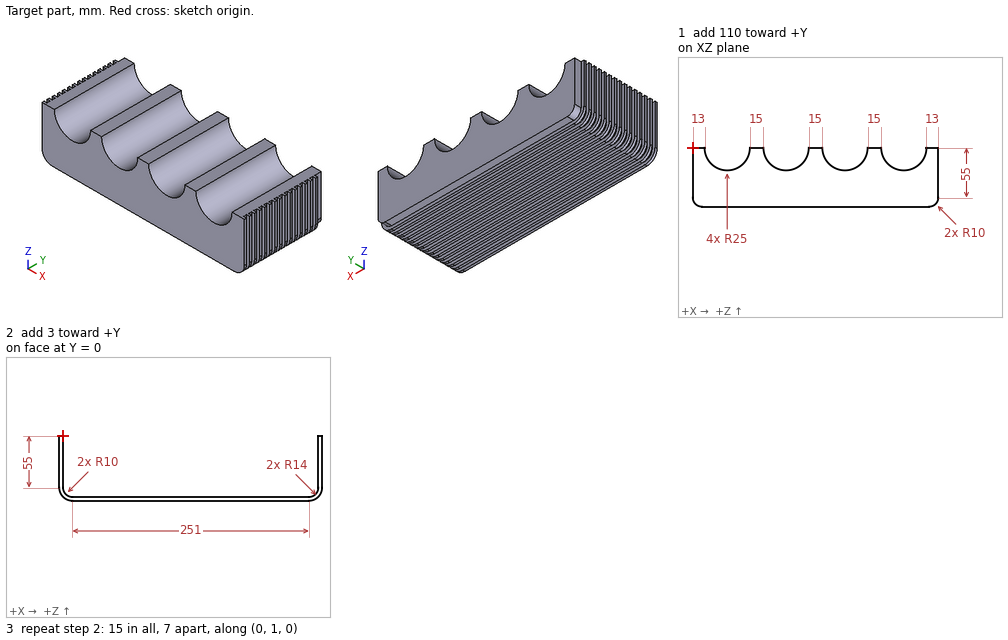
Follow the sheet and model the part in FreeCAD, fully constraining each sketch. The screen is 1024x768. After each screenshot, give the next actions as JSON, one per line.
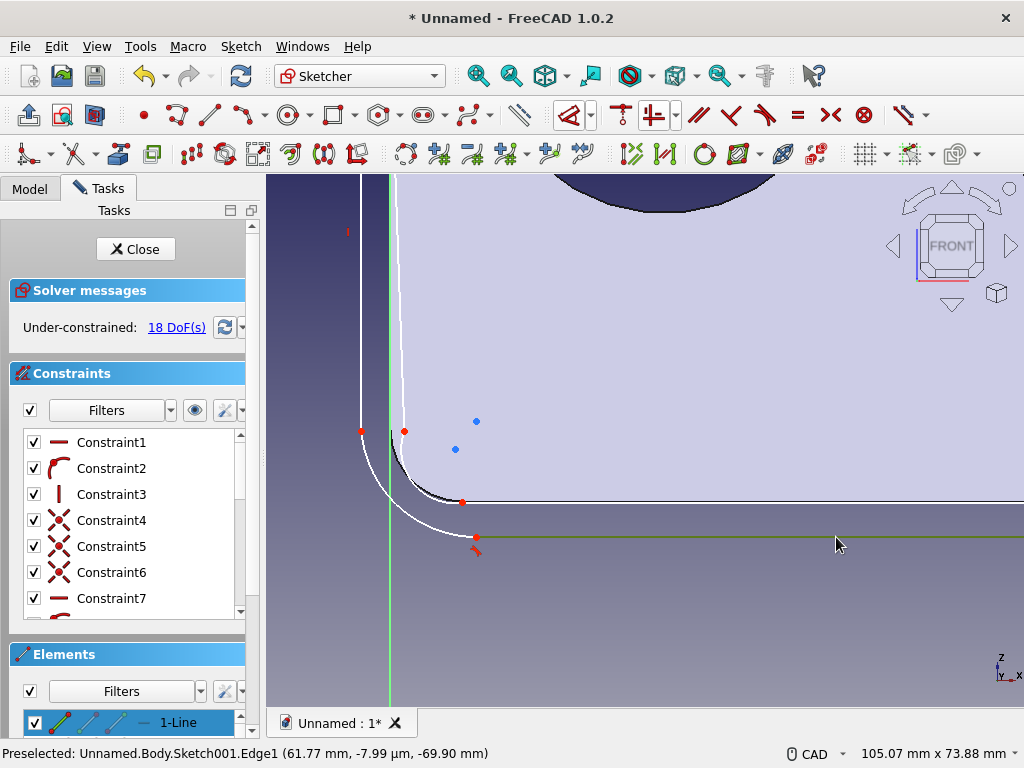
{"action": "scroll", "coordinate": [376, 481], "scroll_direction": "down", "scroll_amount": 8}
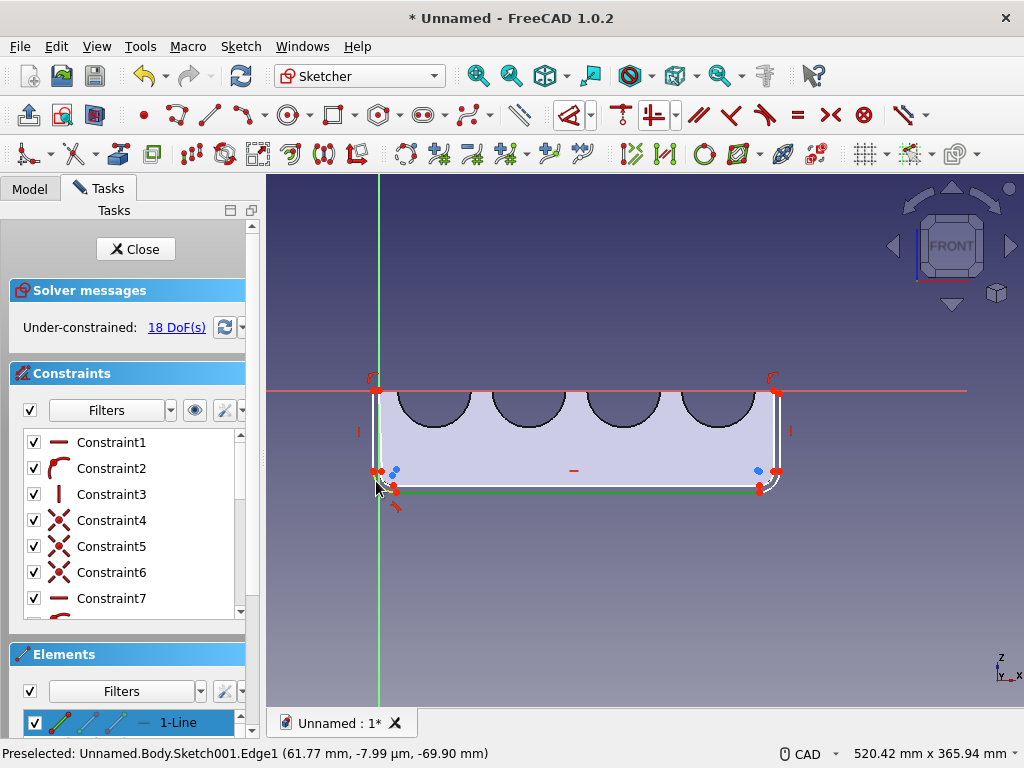
{"action": "scroll", "coordinate": [768, 490], "scroll_direction": "up", "scroll_amount": 5}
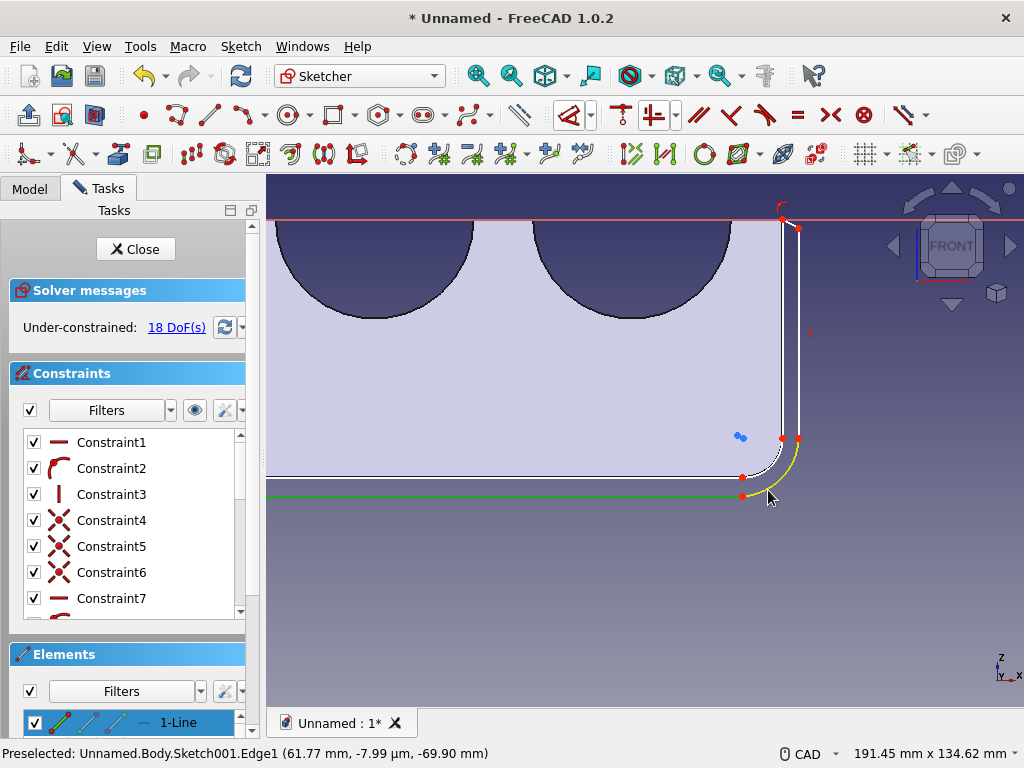
{"action": "left_click", "coordinate": [768, 489]}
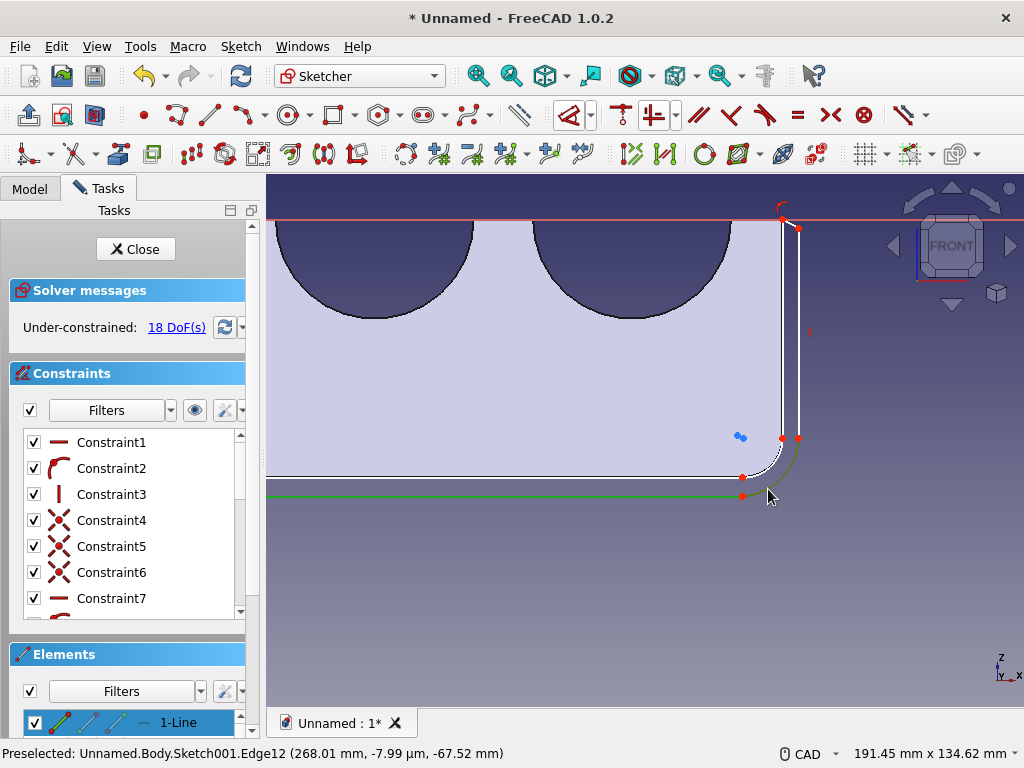
{"action": "left_click", "coordinate": [765, 116]}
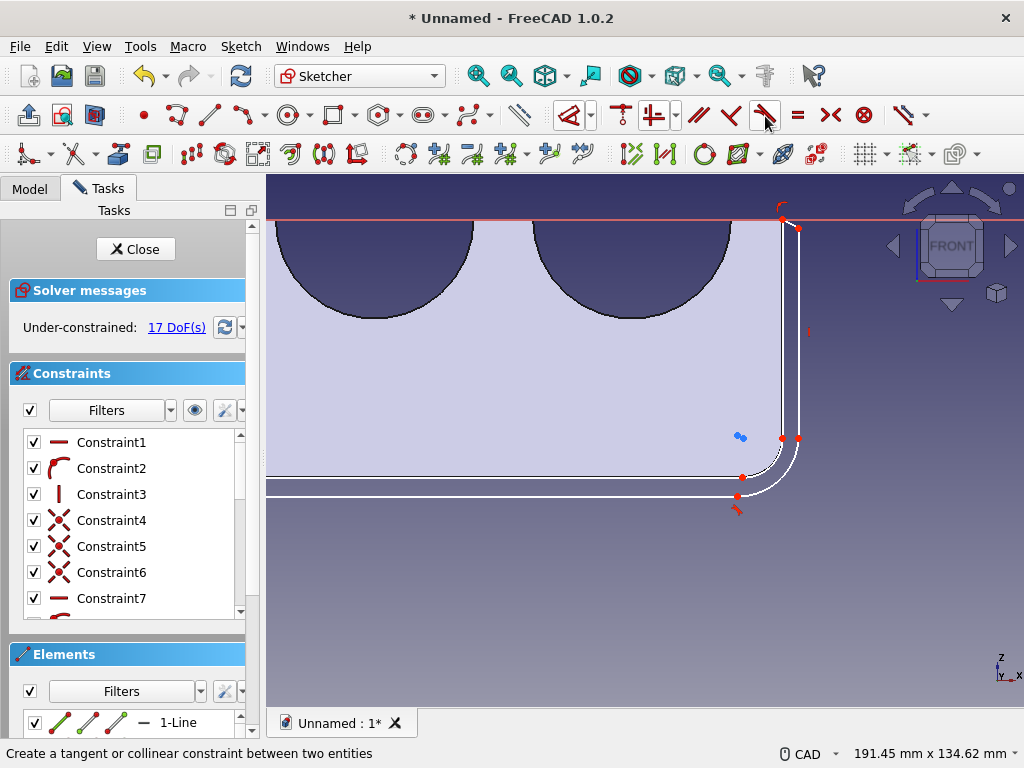
{"action": "scroll", "coordinate": [769, 489], "scroll_direction": "down", "scroll_amount": 5}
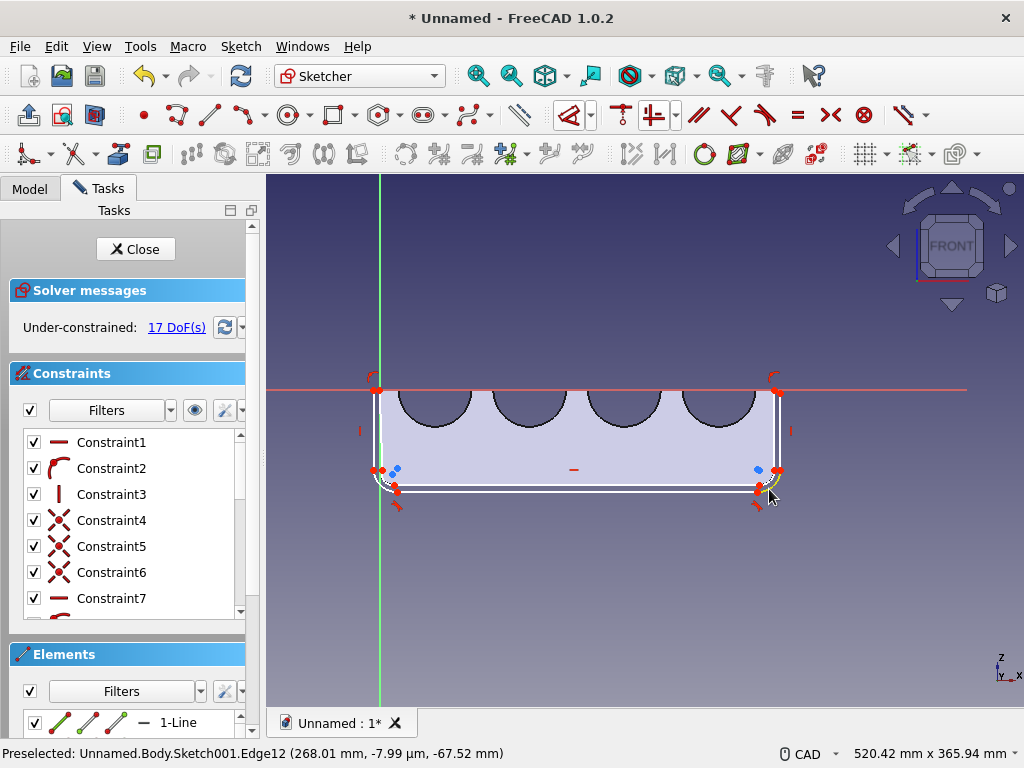
{"action": "scroll", "coordinate": [374, 447], "scroll_direction": "up", "scroll_amount": 5}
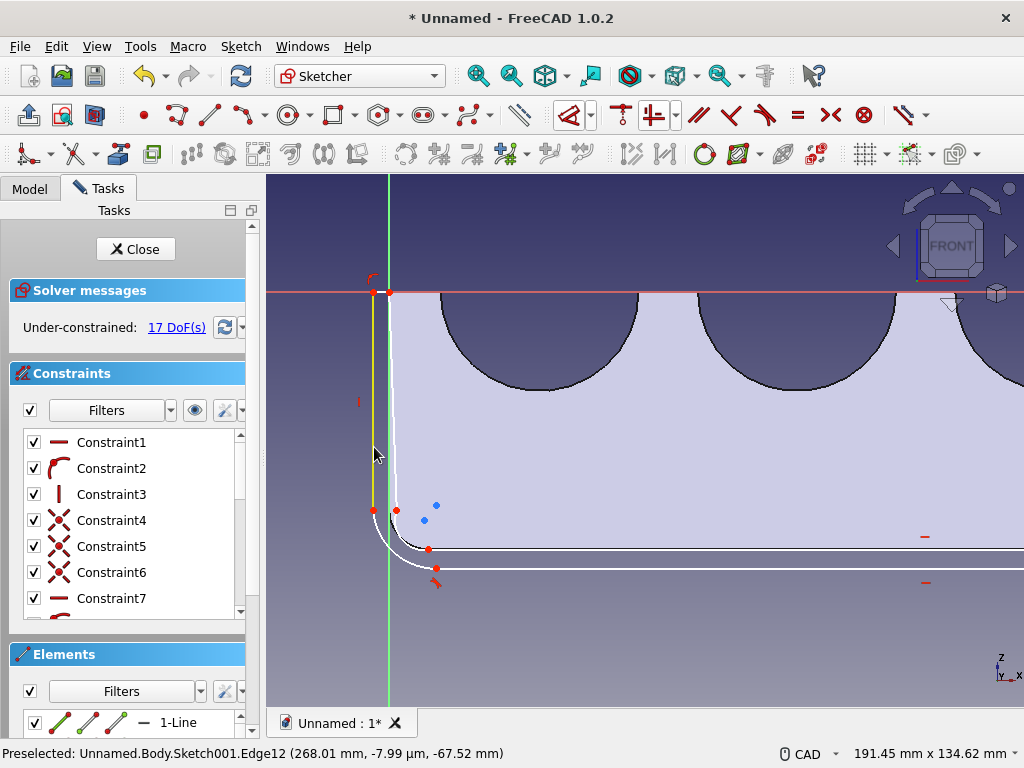
{"action": "left_click", "coordinate": [373, 445]}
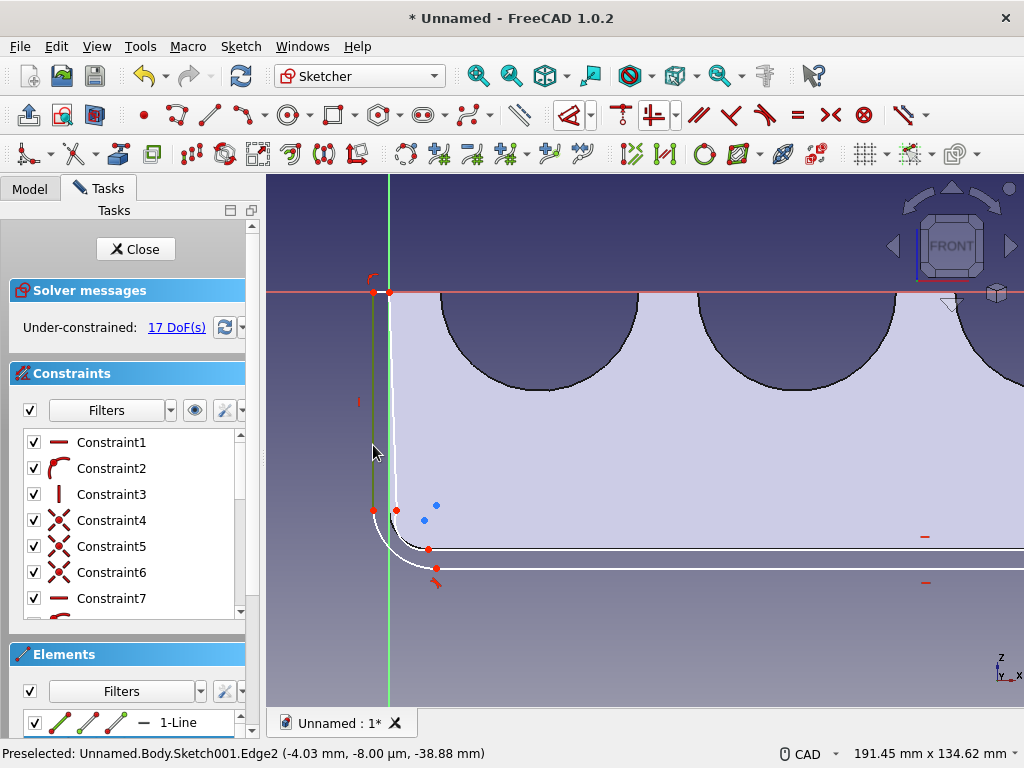
{"action": "left_click", "coordinate": [409, 563]}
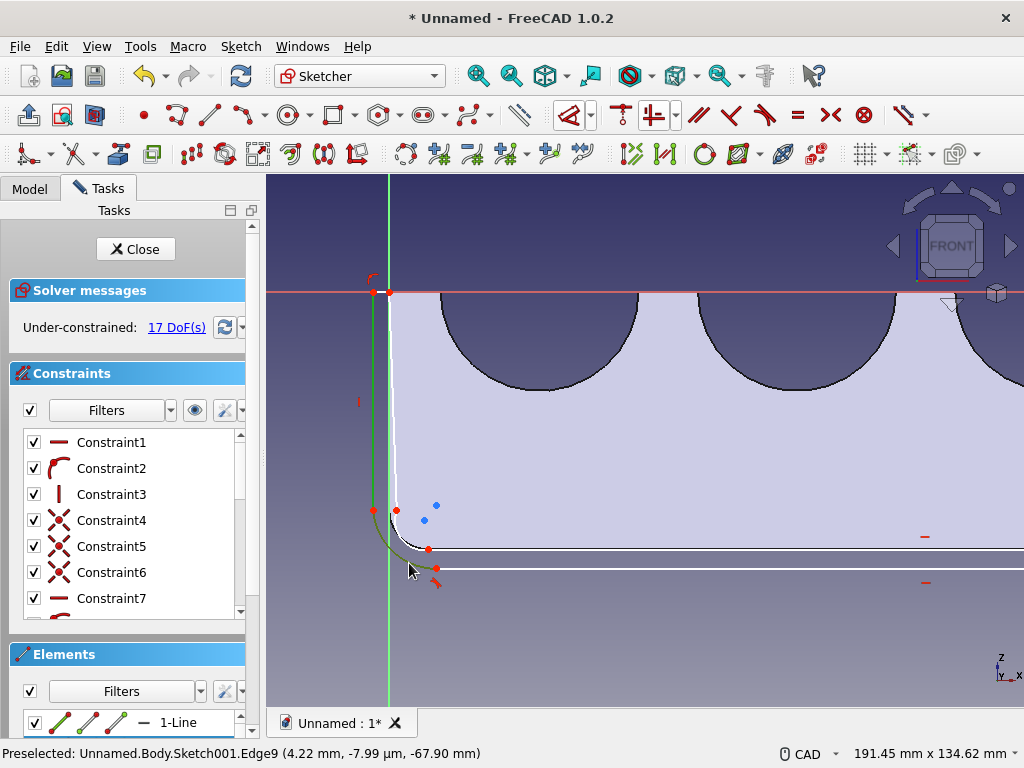
{"action": "left_click", "coordinate": [765, 116]}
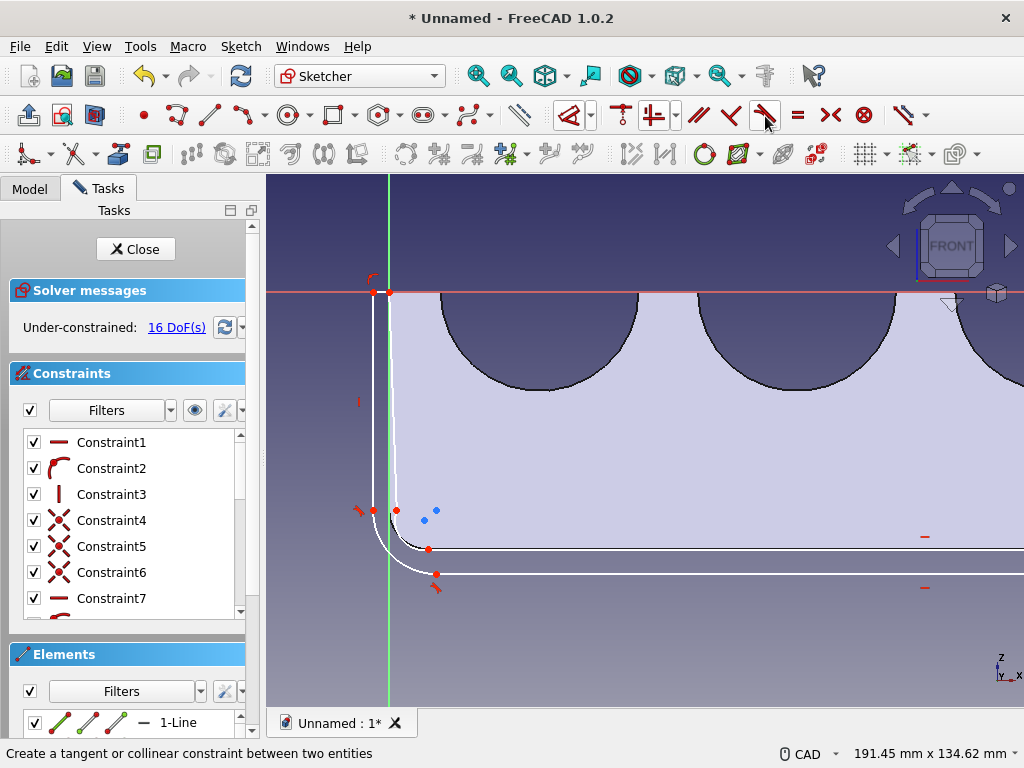
{"action": "left_click", "coordinate": [391, 358]}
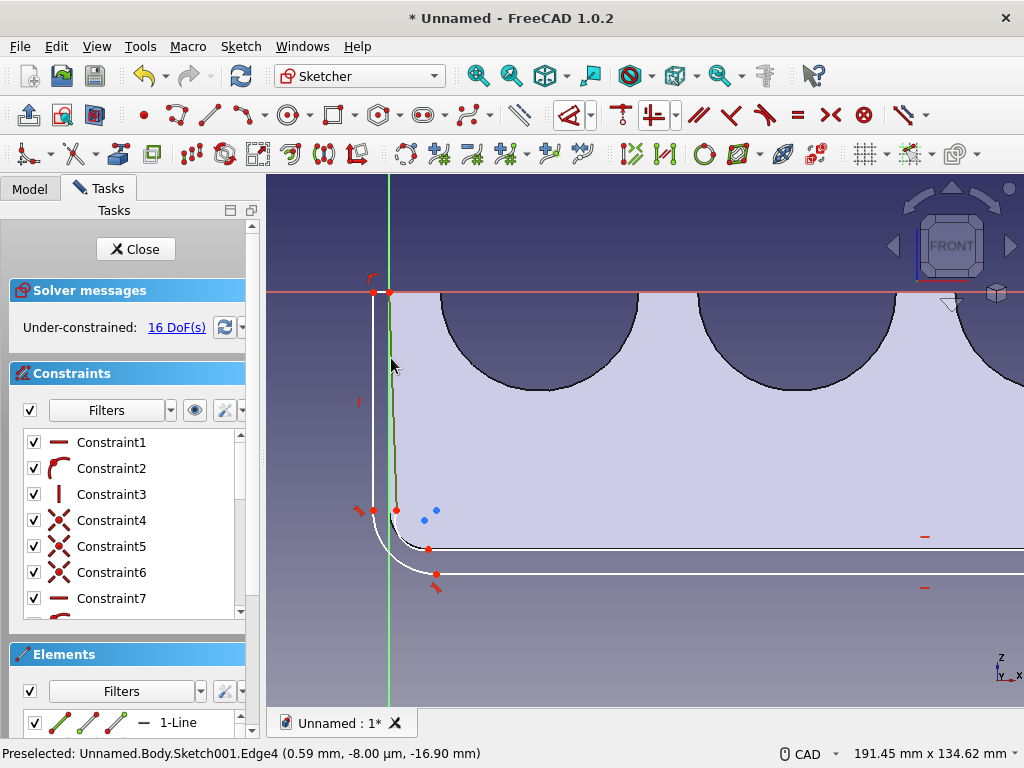
{"action": "left_click", "coordinate": [411, 547]}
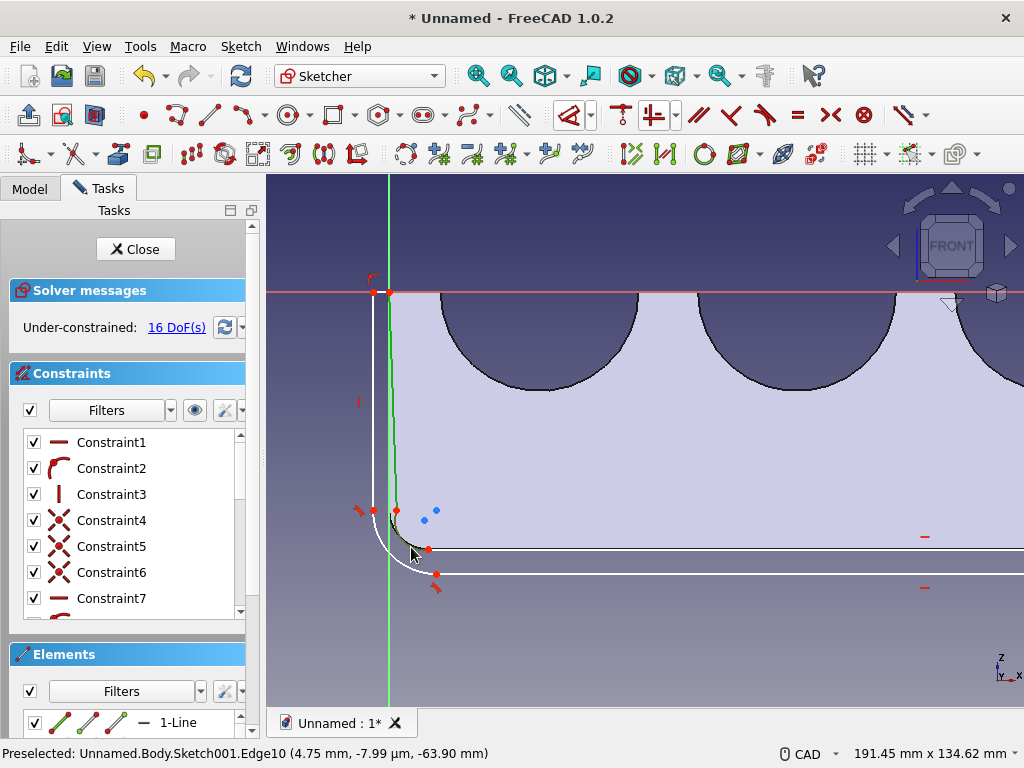
{"action": "left_click", "coordinate": [765, 116]}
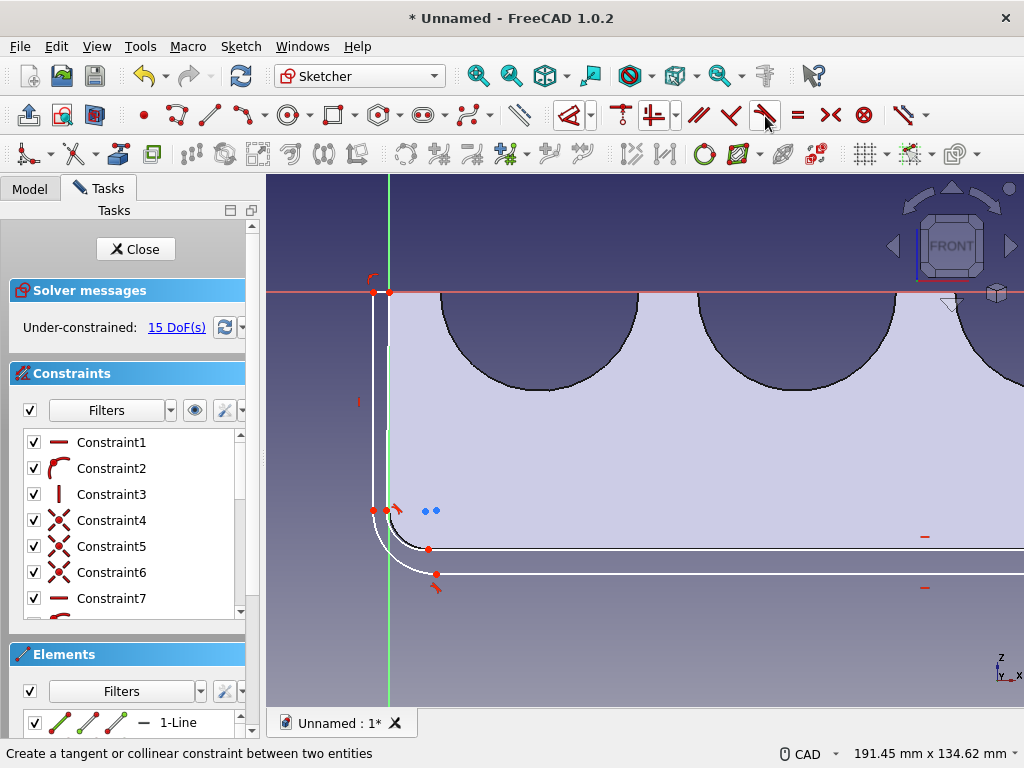
{"action": "left_click", "coordinate": [727, 550]}